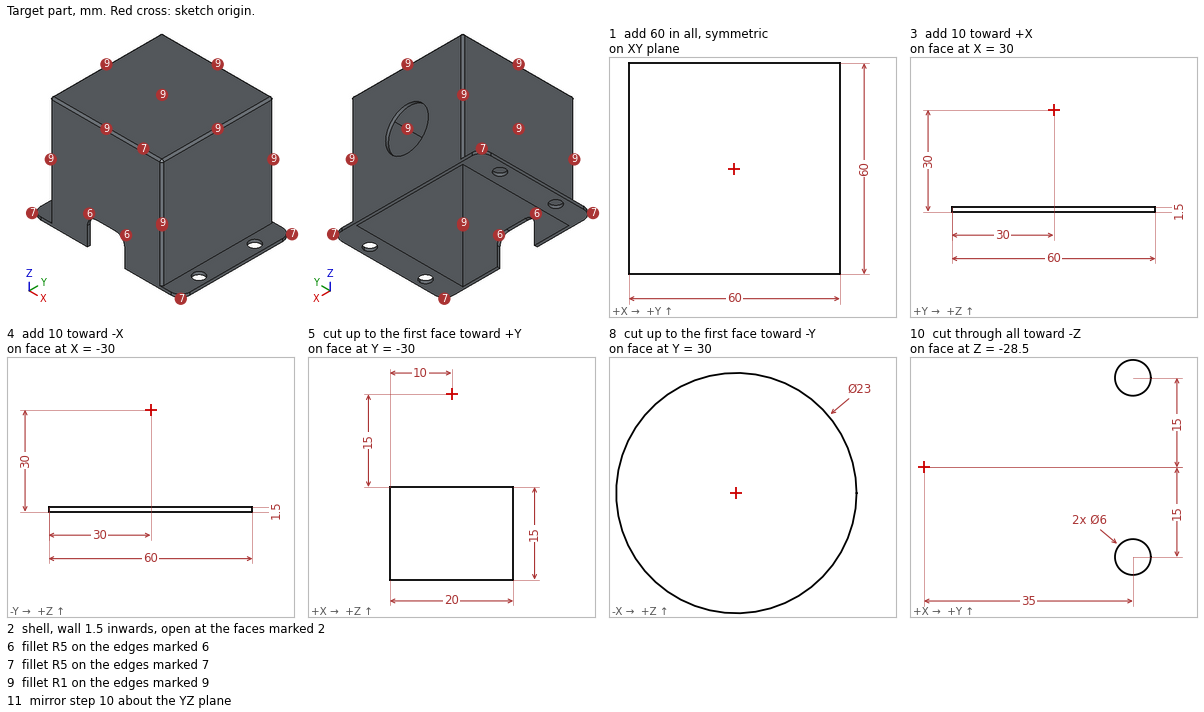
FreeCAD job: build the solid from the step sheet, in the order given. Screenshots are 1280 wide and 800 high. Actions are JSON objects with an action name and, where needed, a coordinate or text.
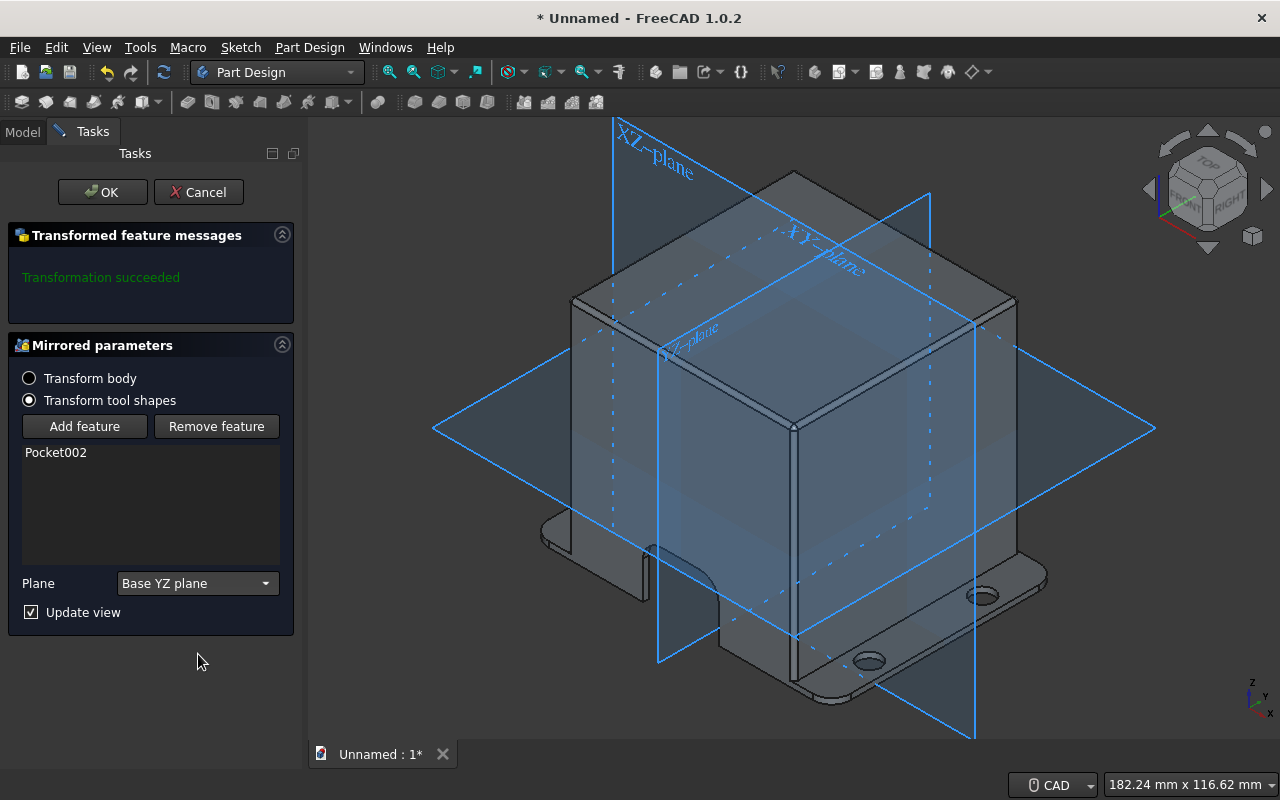
{"action": "left_click", "coordinate": [103, 192]}